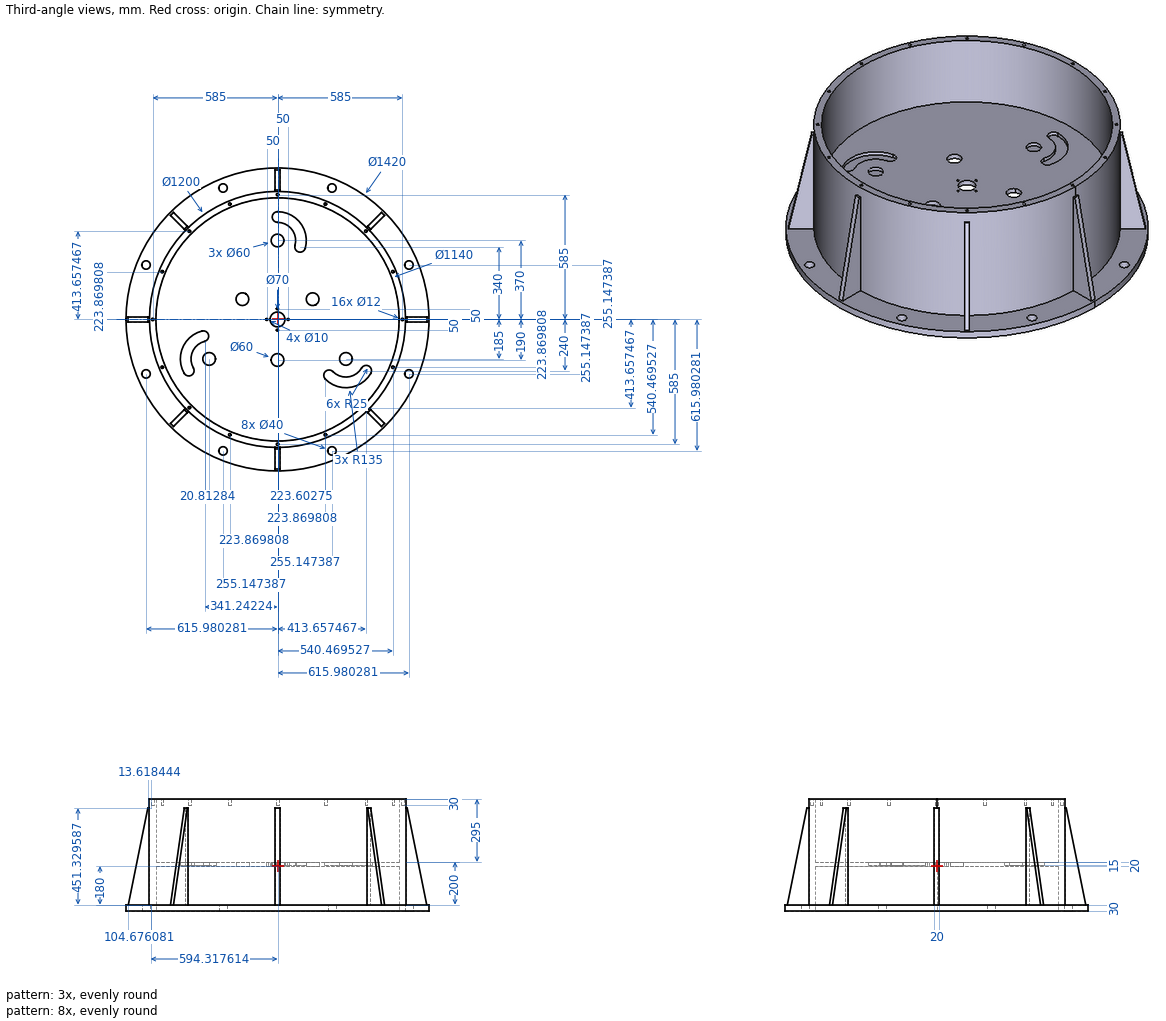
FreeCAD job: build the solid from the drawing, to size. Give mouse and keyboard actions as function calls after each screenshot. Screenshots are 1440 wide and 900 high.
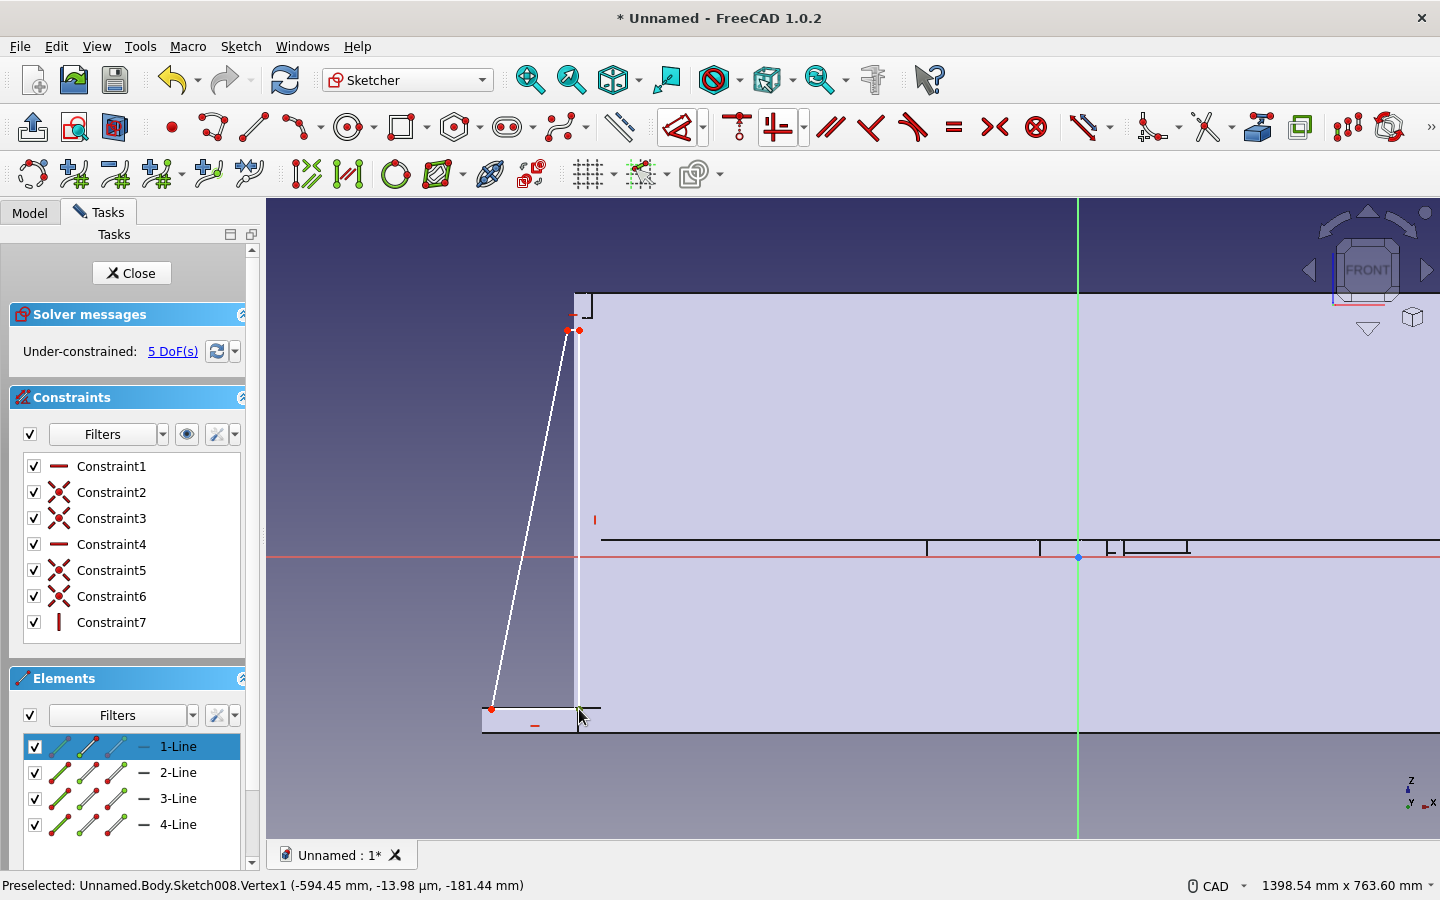
click(702, 128)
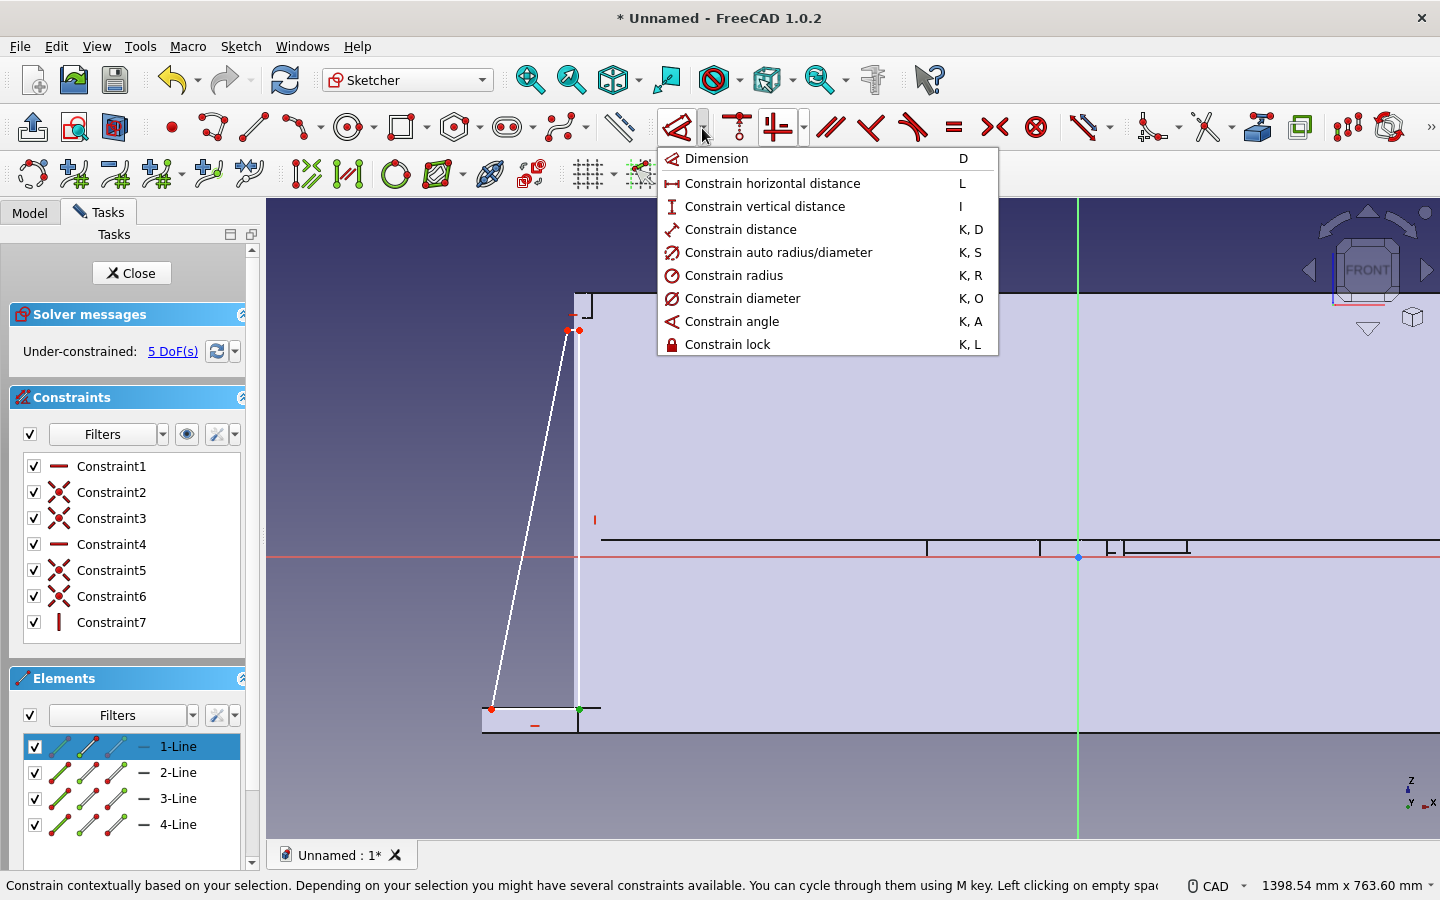
click(828, 206)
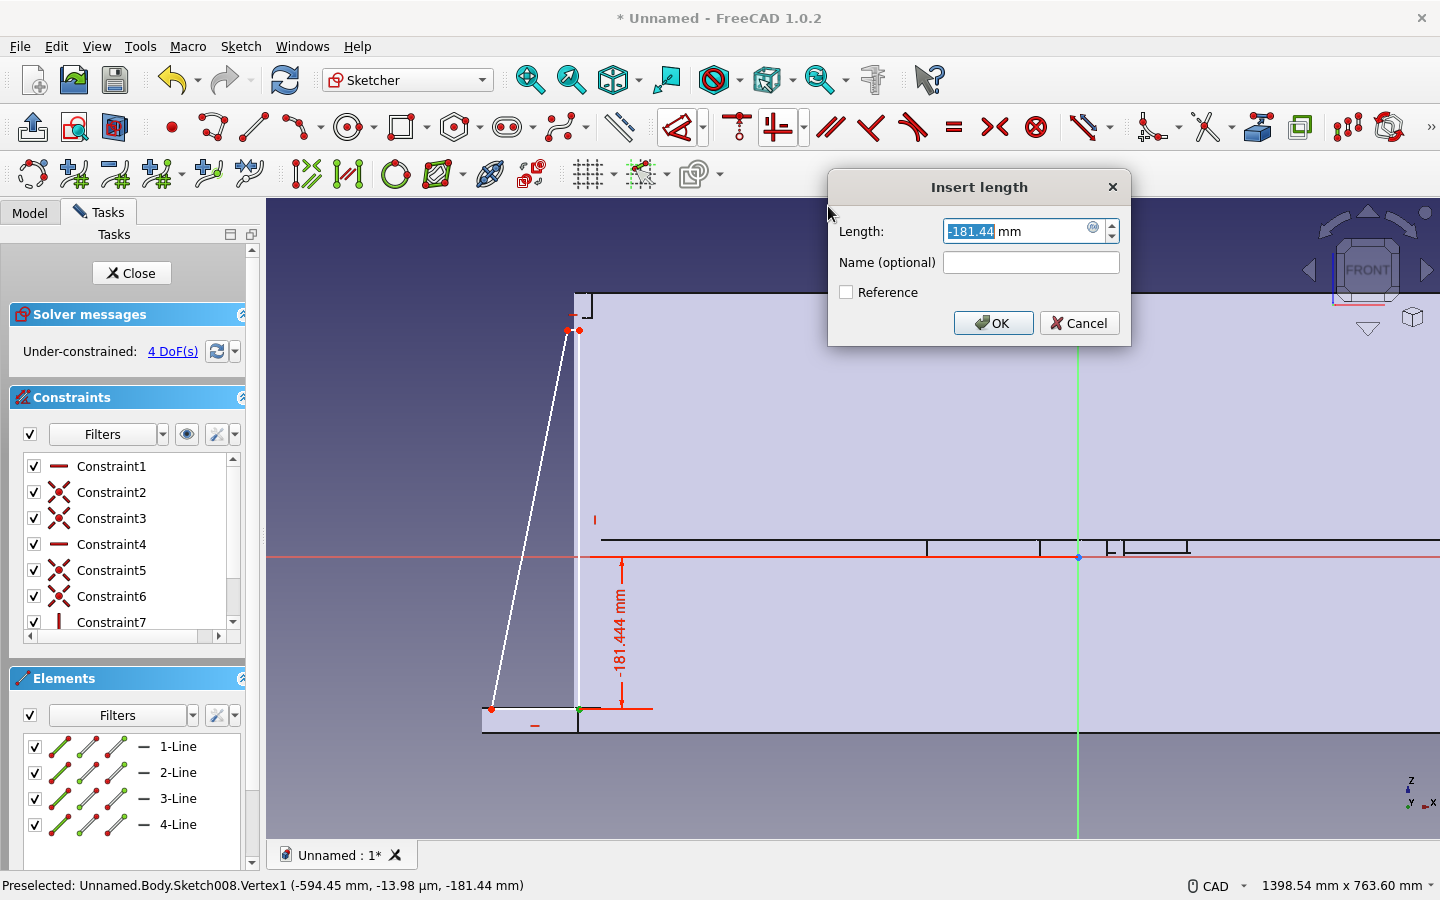
text(-180)
key(Return)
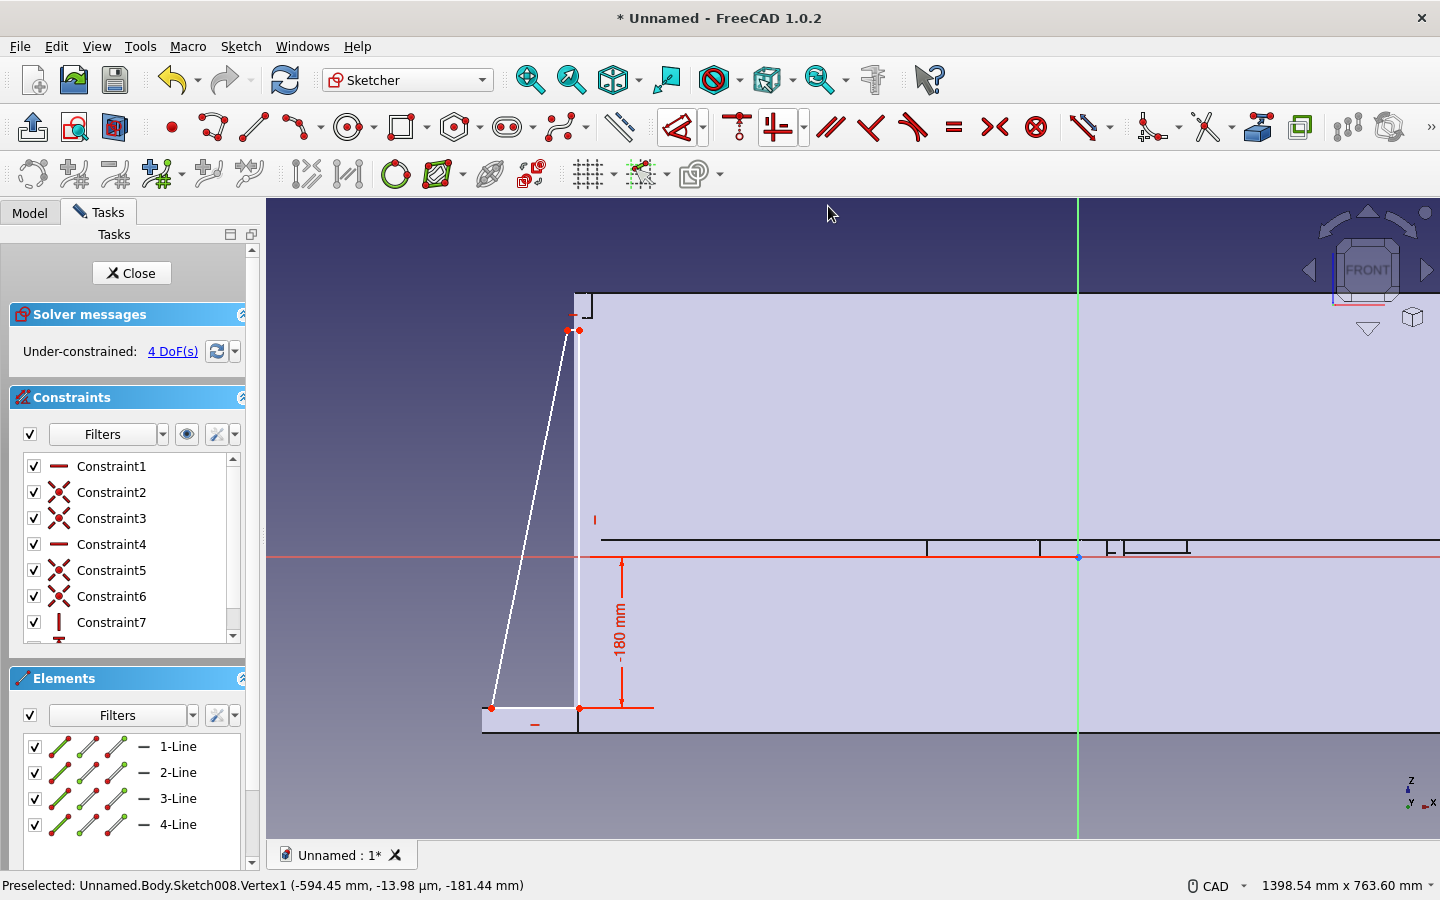
scroll(573, 330, up, 7)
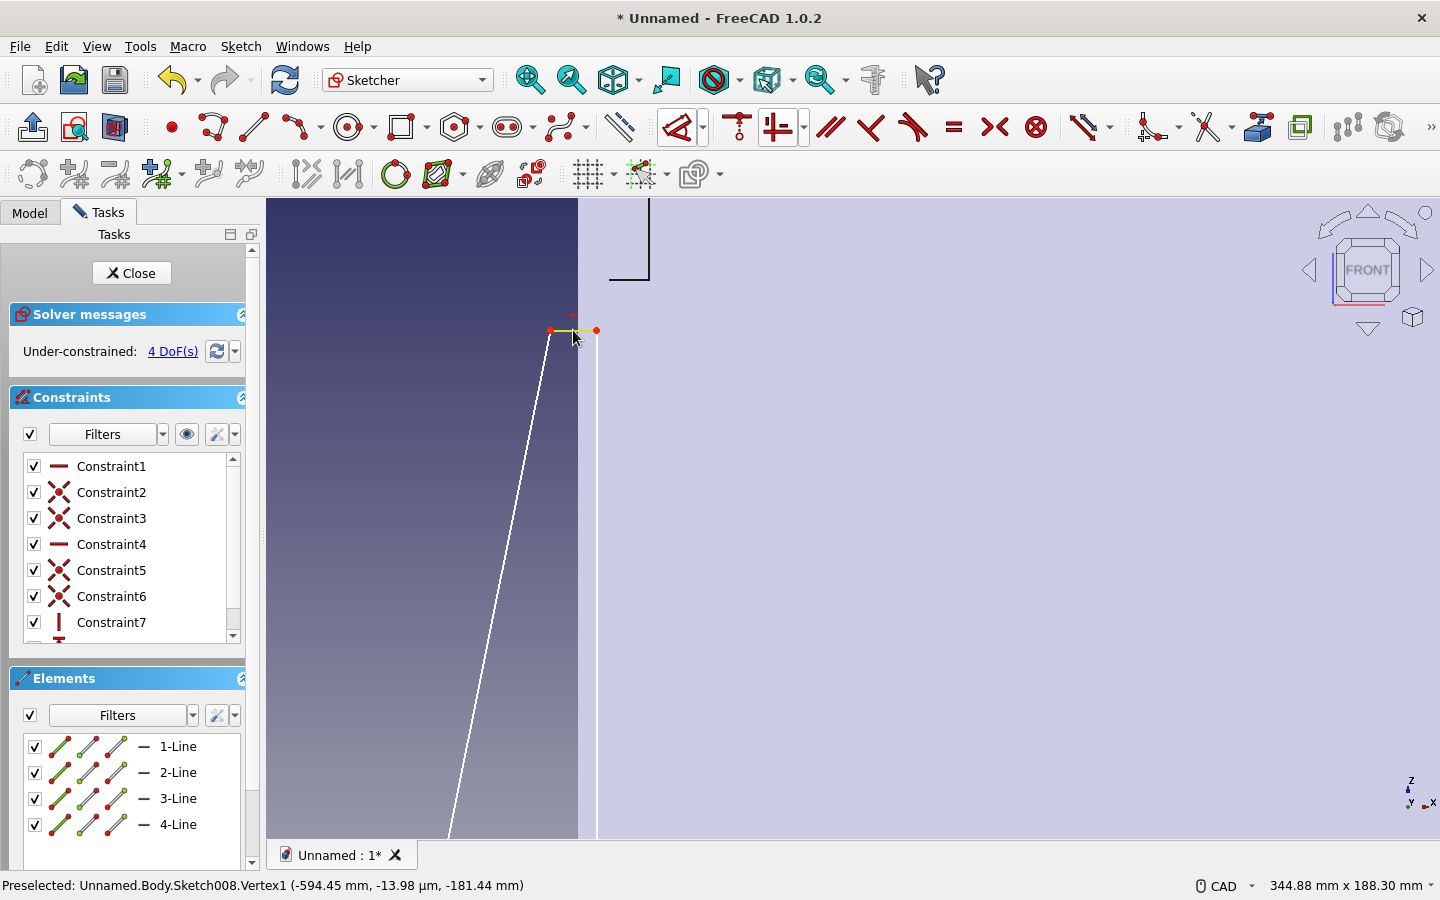
click(574, 331)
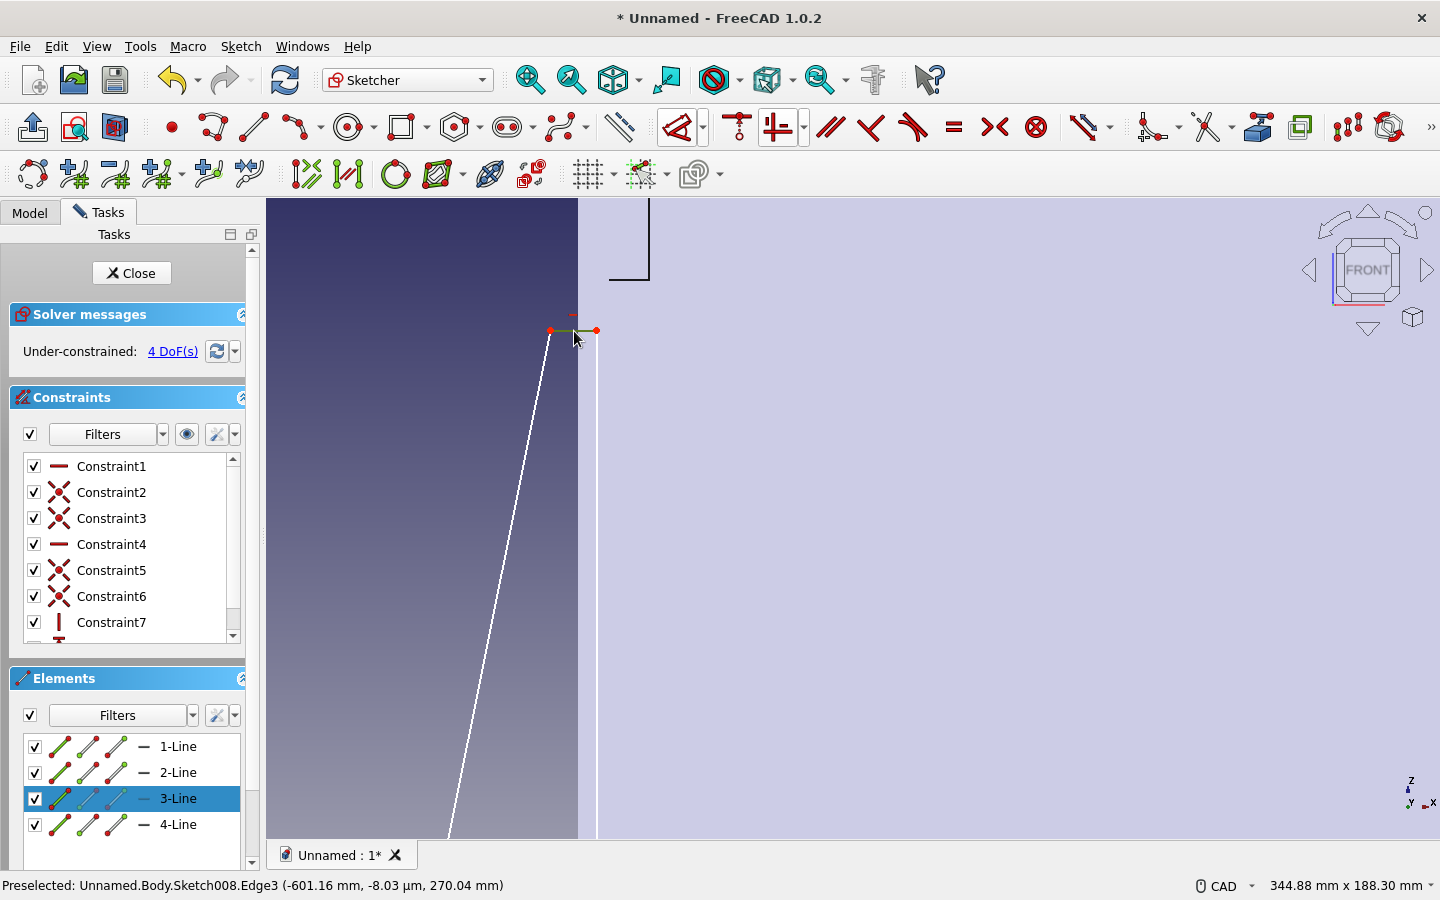
key(l)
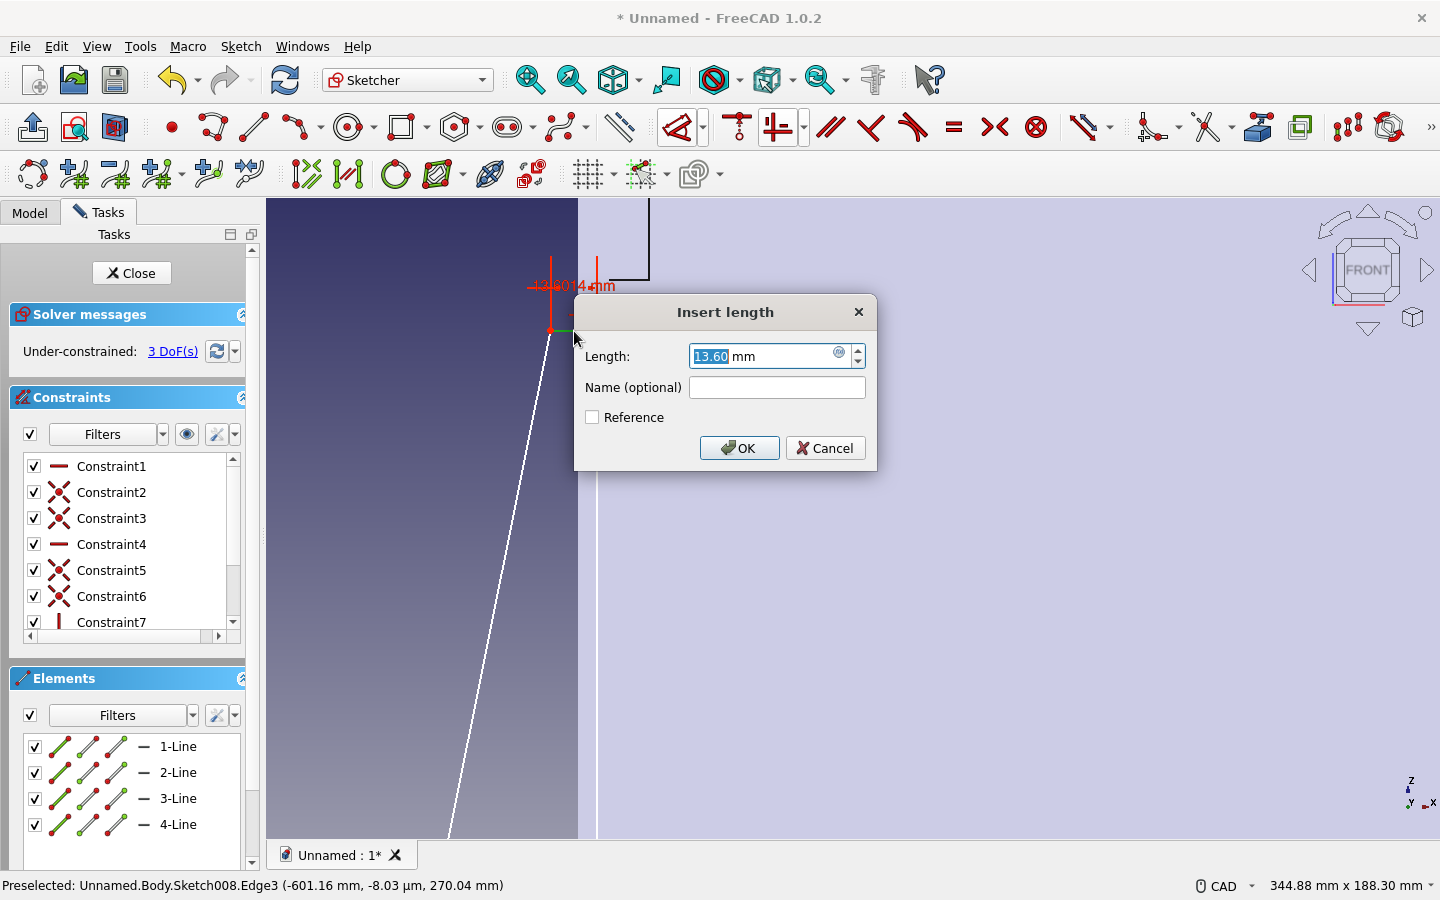
text(13.618444)
key(Return)